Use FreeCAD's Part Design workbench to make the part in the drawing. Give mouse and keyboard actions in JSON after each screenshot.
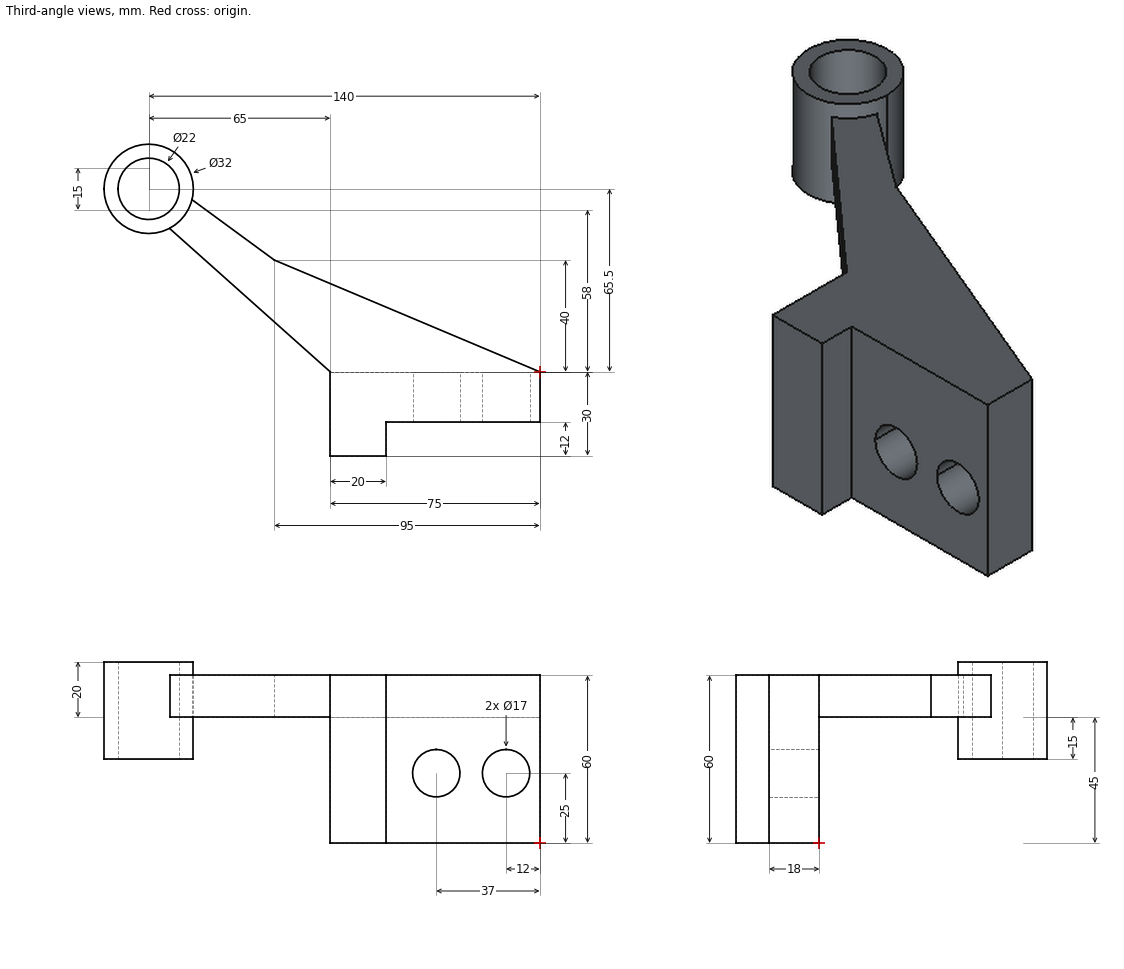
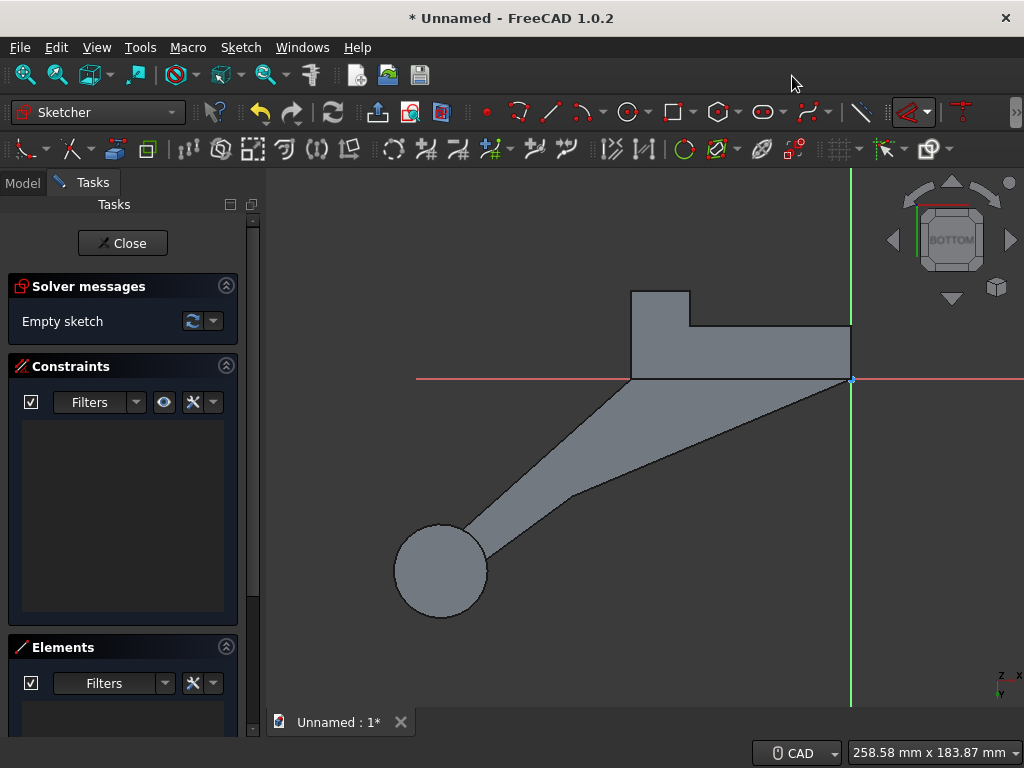
{"action": "scroll", "coordinate": [406, 605], "scroll_direction": "up", "scroll_amount": 8}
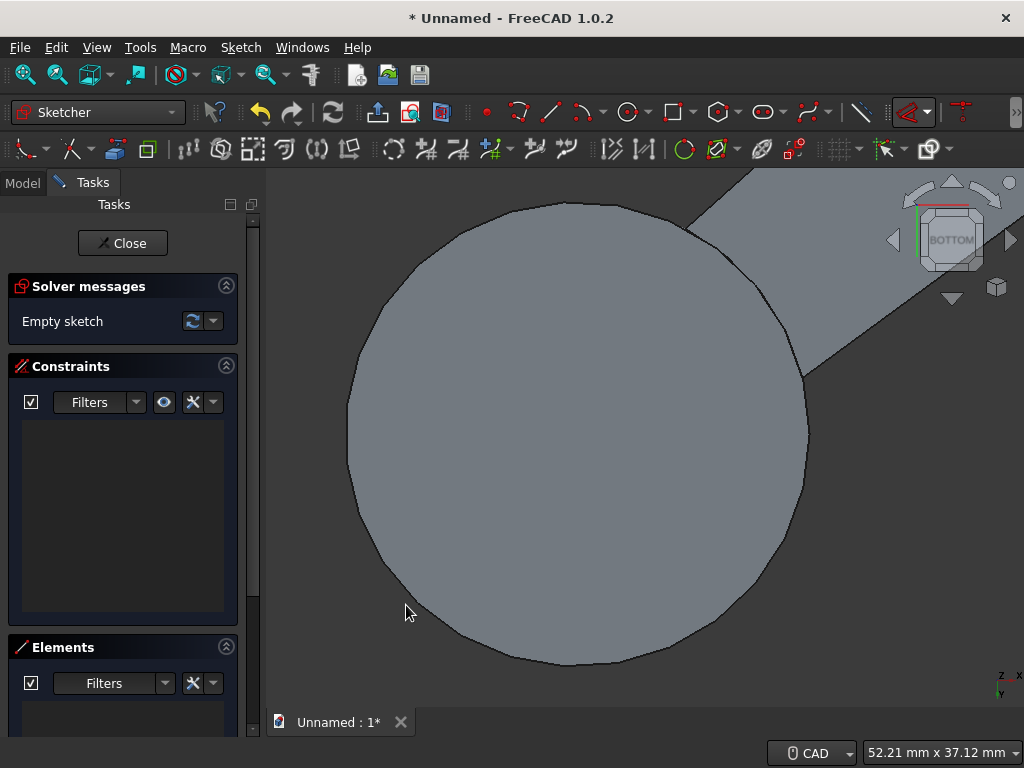
{"action": "left_click", "coordinate": [628, 112]}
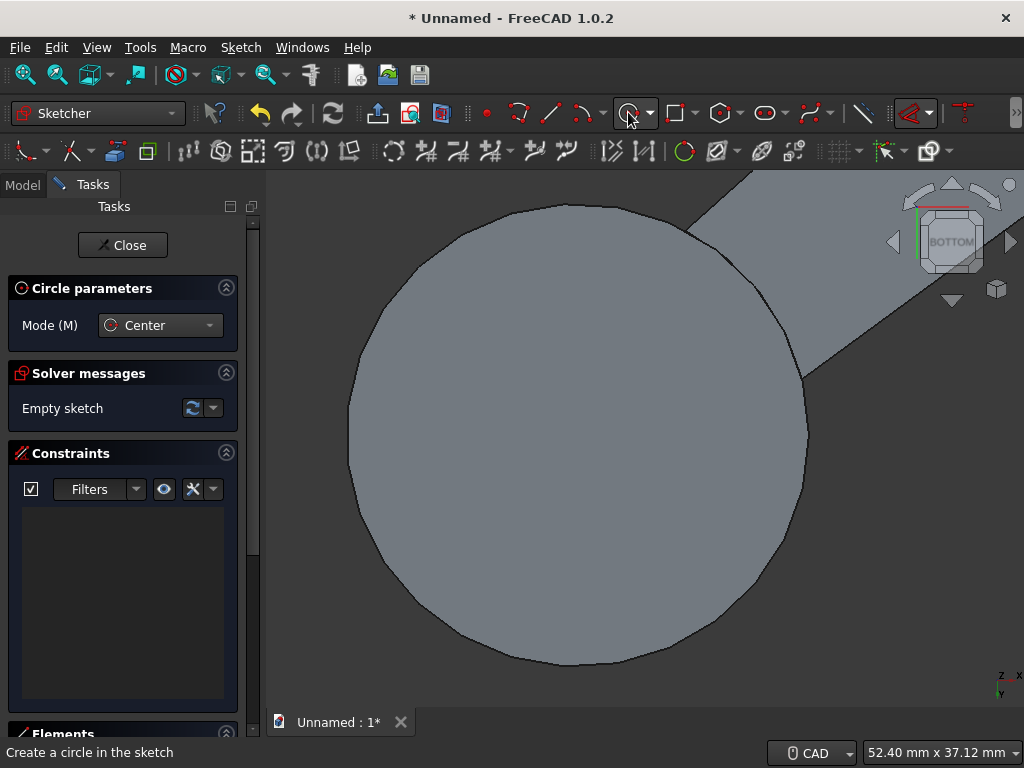
{"action": "left_click", "coordinate": [578, 435]}
{"action": "left_click", "coordinate": [690, 323]}
{"action": "key", "text": "Escape"}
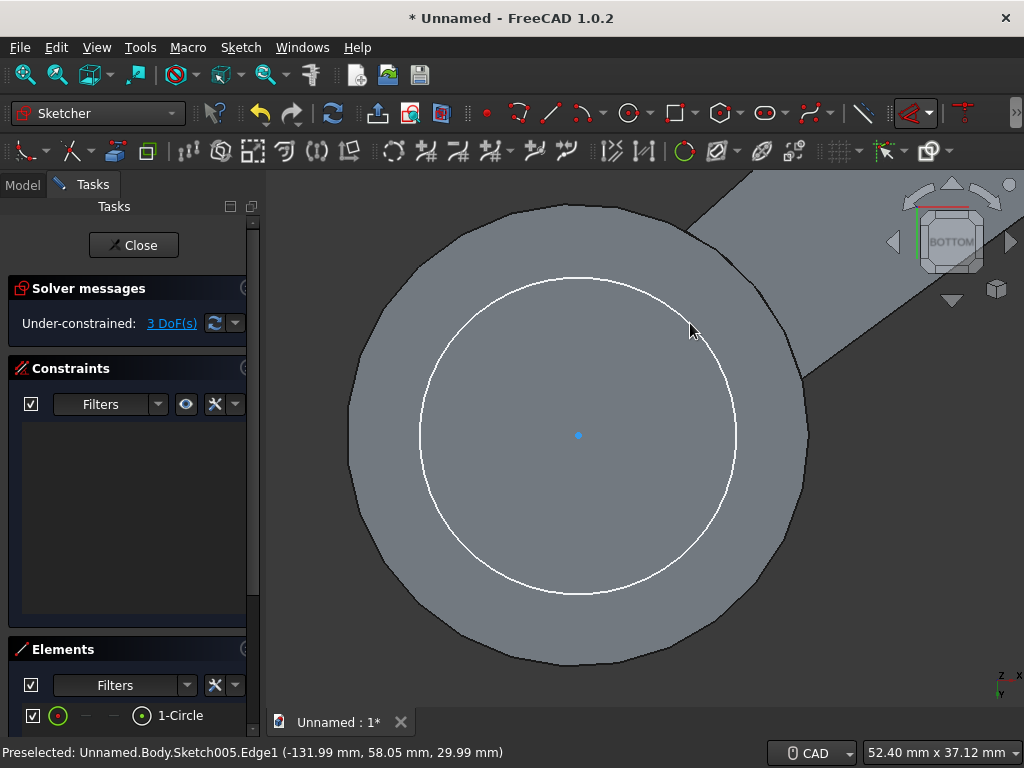
{"action": "left_click", "coordinate": [690, 324]}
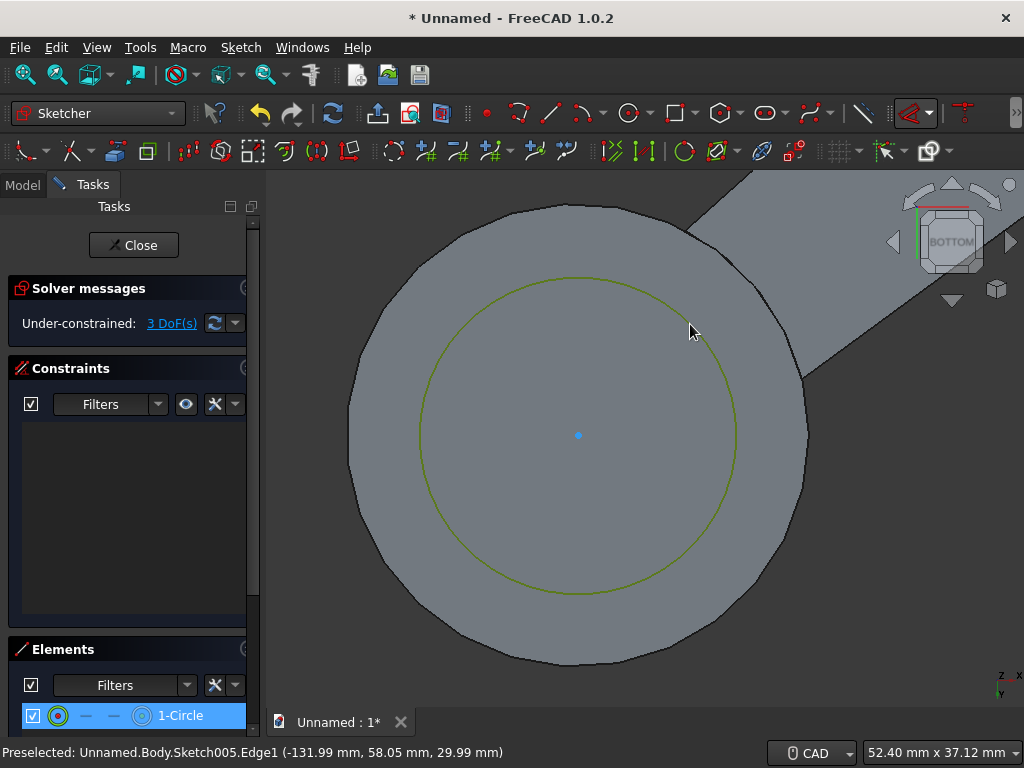
{"action": "key", "text": "k o"}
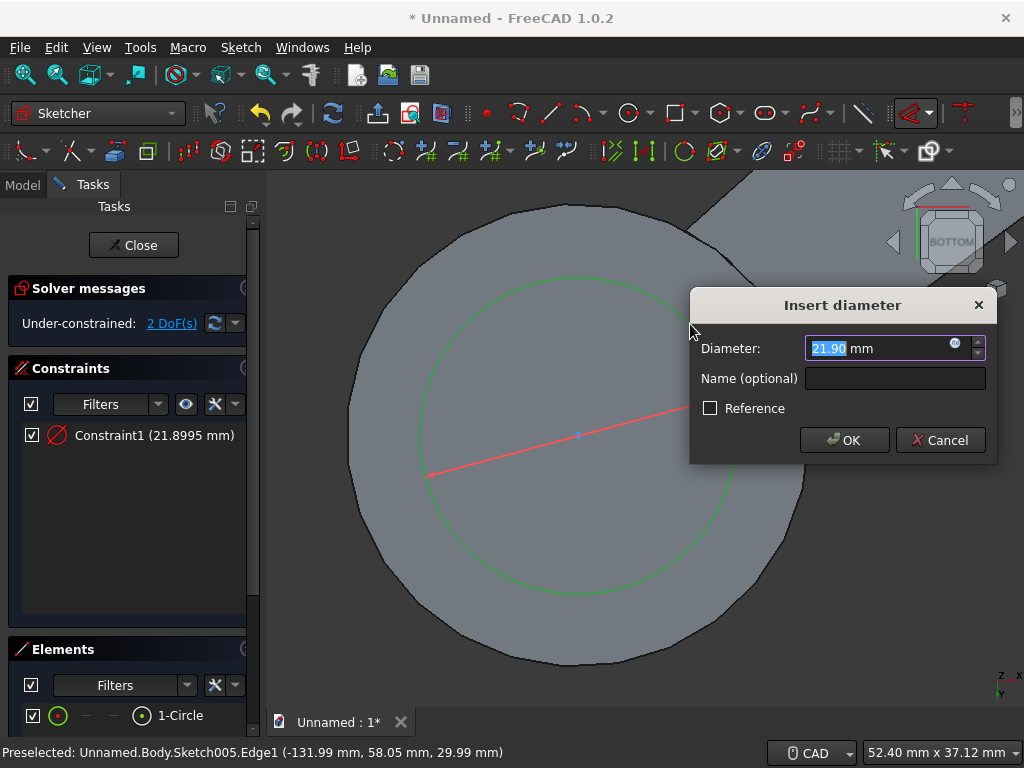
{"action": "type", "text": "22"}
{"action": "key", "text": "Return"}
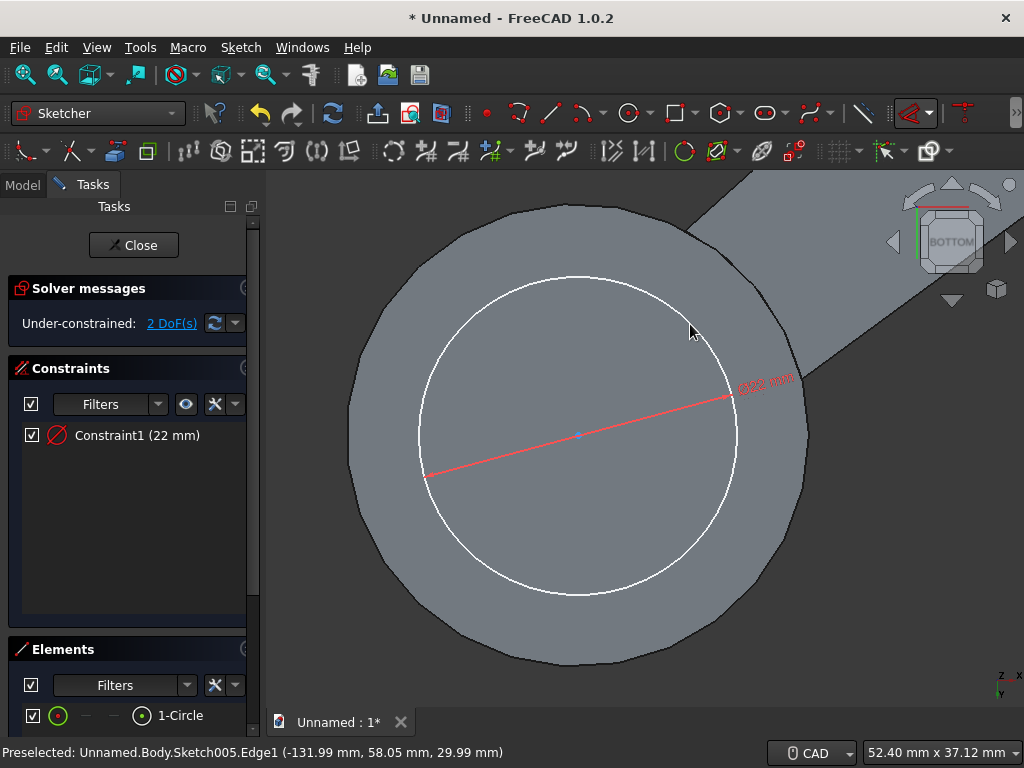
{"action": "left_click", "coordinate": [578, 436]}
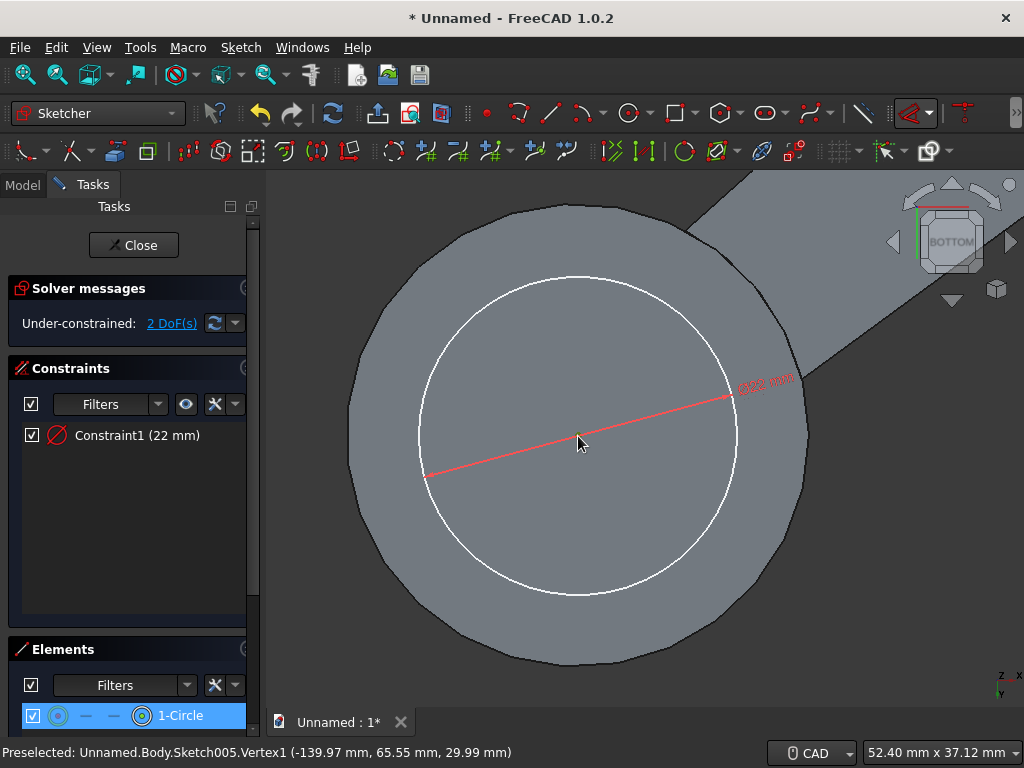
{"action": "left_click", "coordinate": [932, 114]}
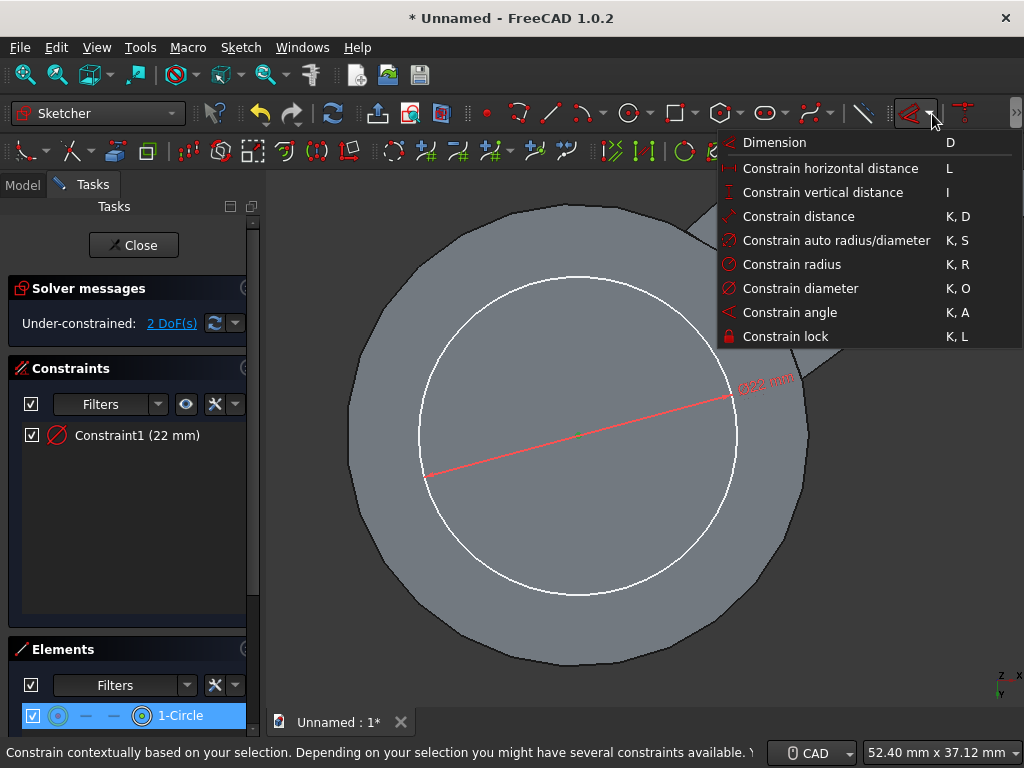
{"action": "left_click", "coordinate": [870, 168]}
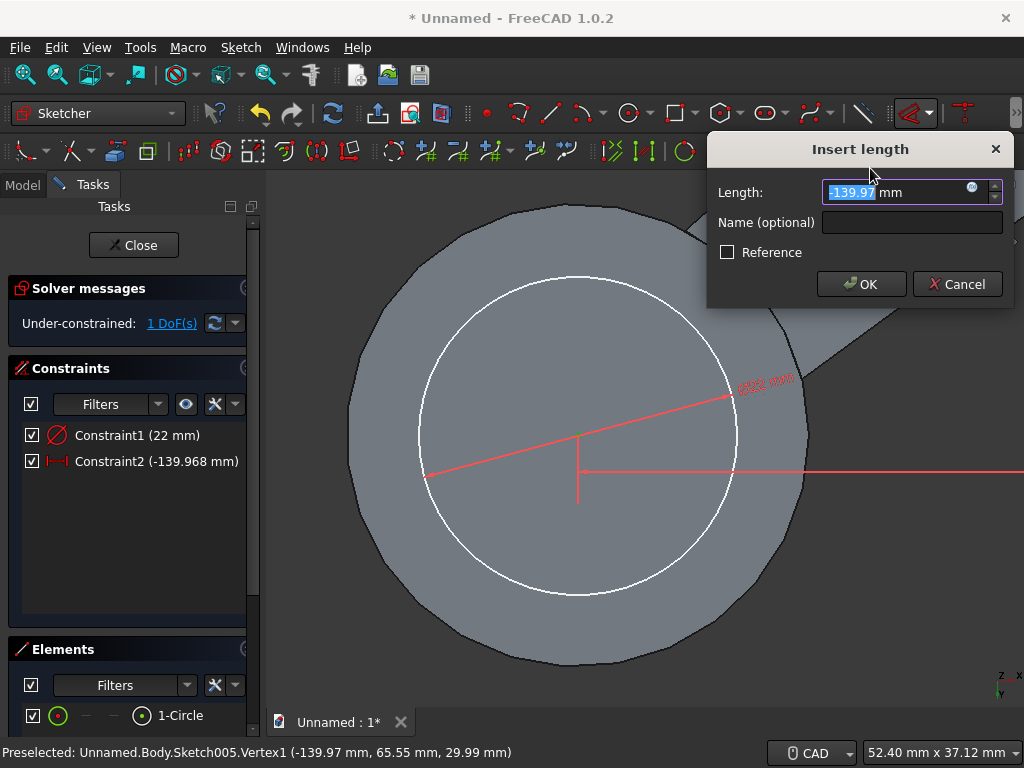
{"action": "type", "text": "-140"}
{"action": "key", "text": "Return"}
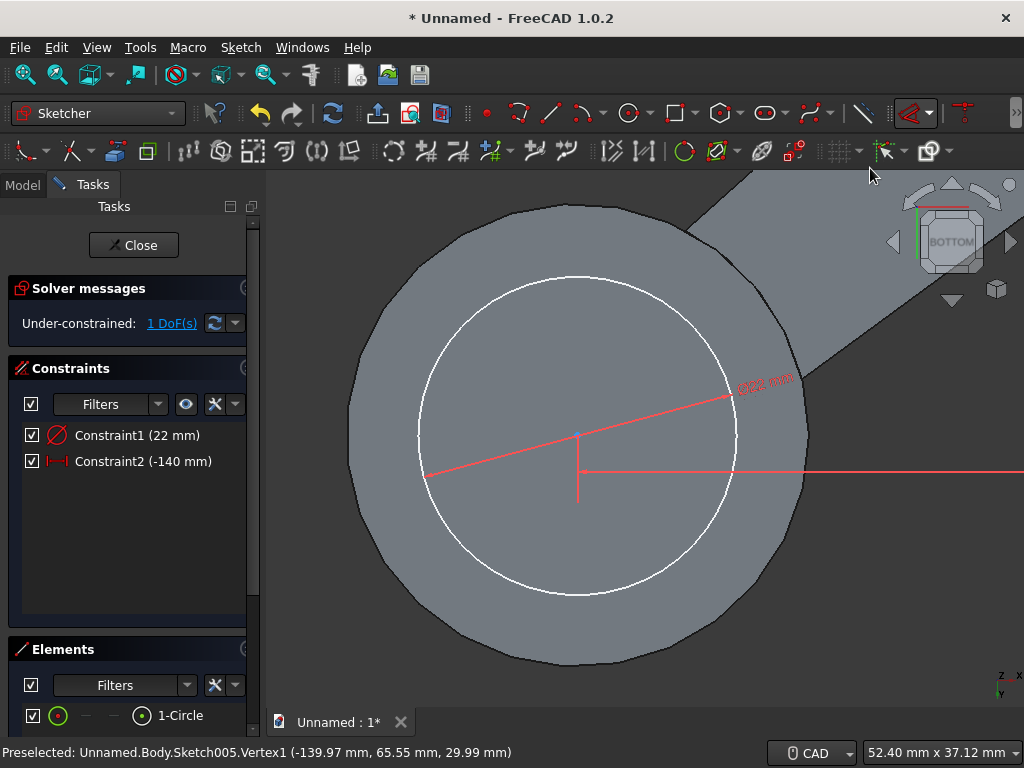
{"action": "left_click", "coordinate": [578, 436]}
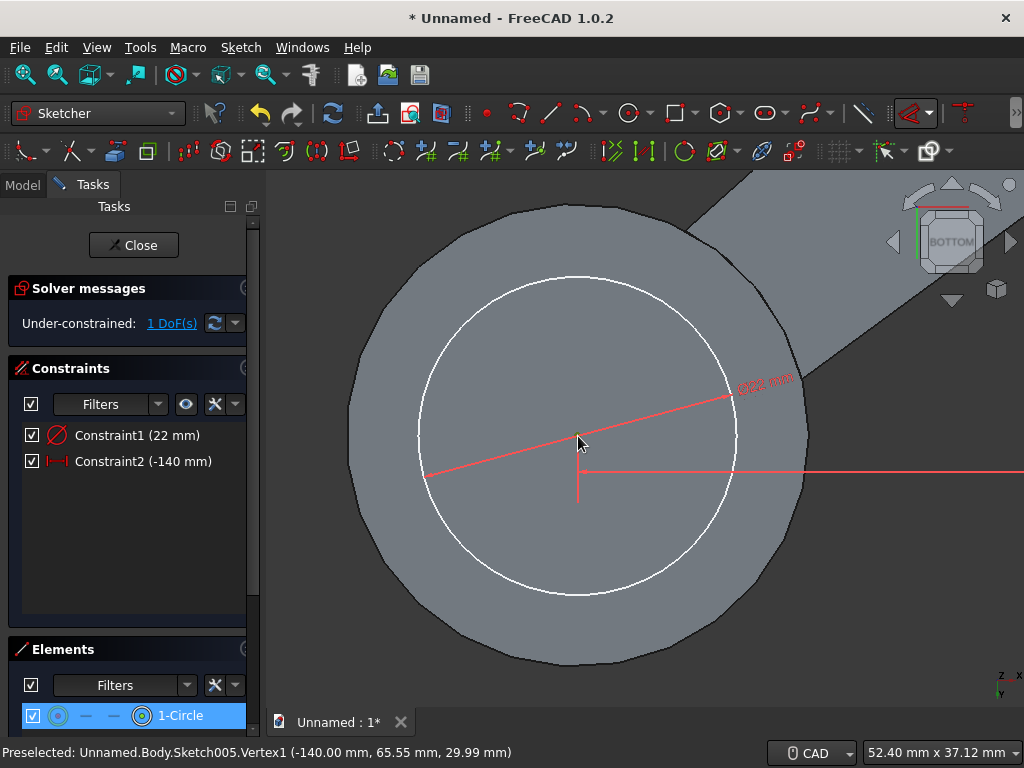
{"action": "left_click", "coordinate": [932, 114]}